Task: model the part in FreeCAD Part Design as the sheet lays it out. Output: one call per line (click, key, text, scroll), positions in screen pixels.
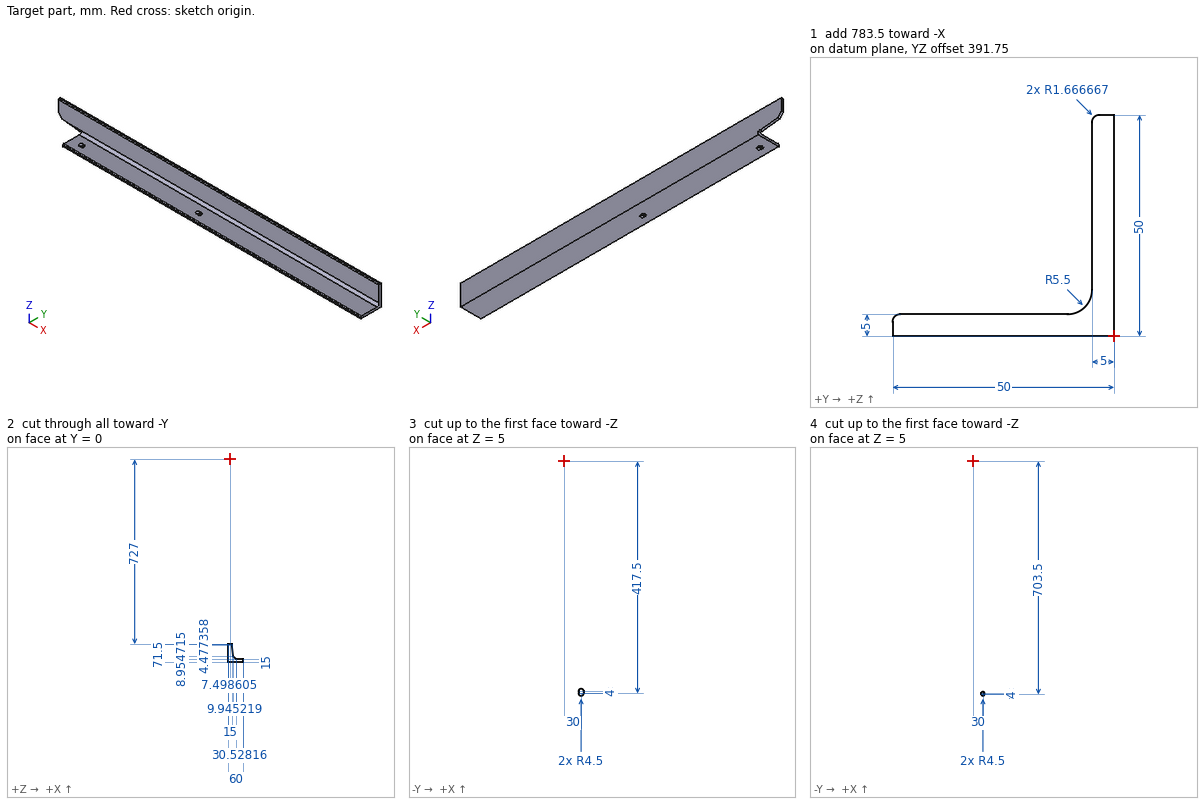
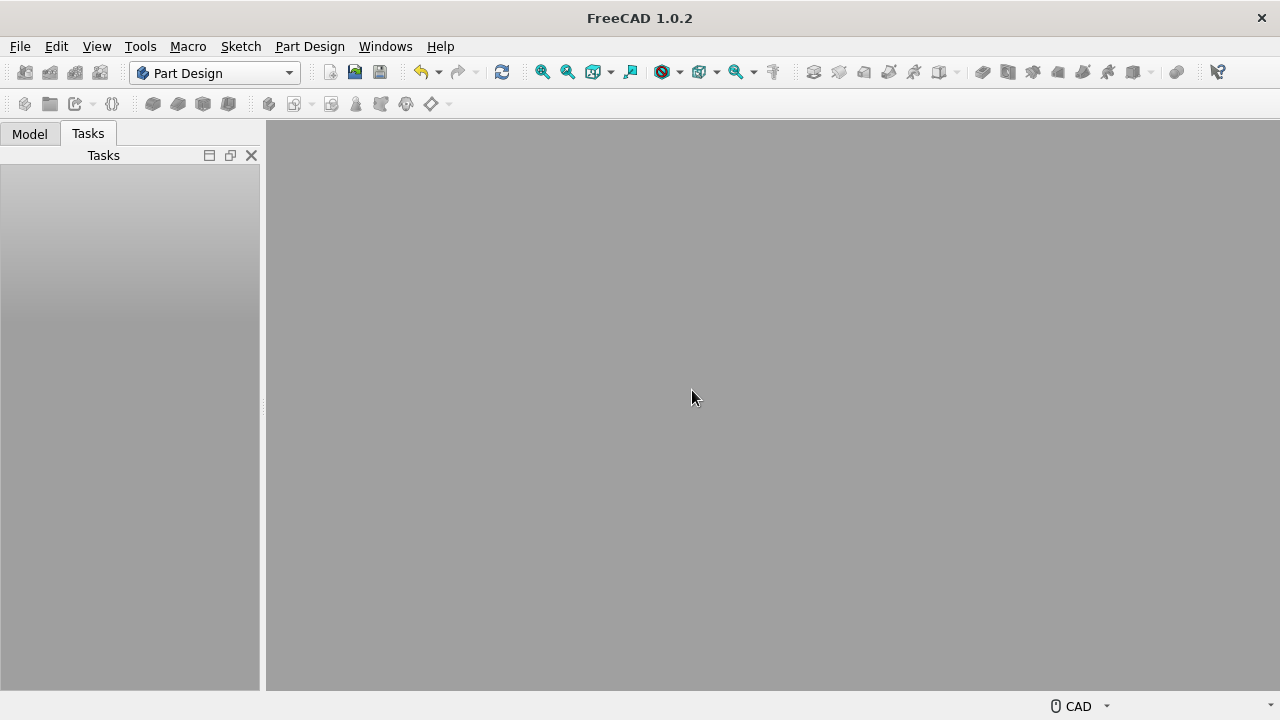
key(ctrl+n)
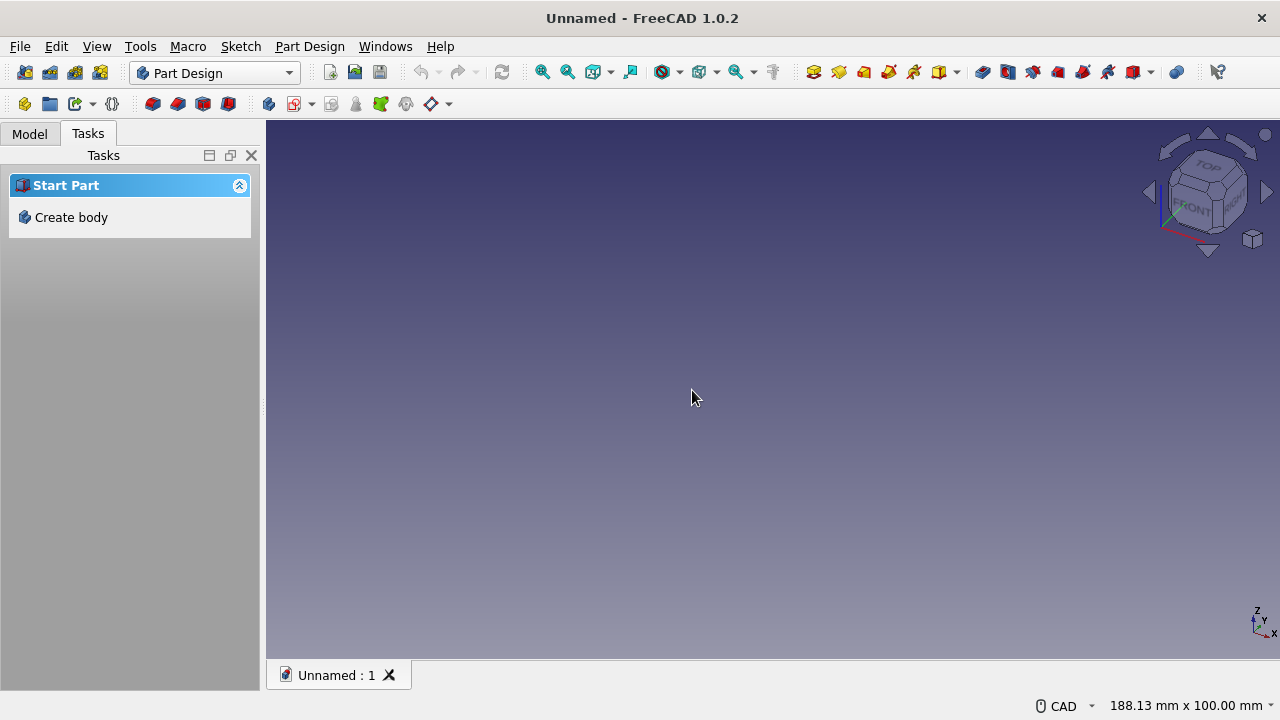
click(269, 104)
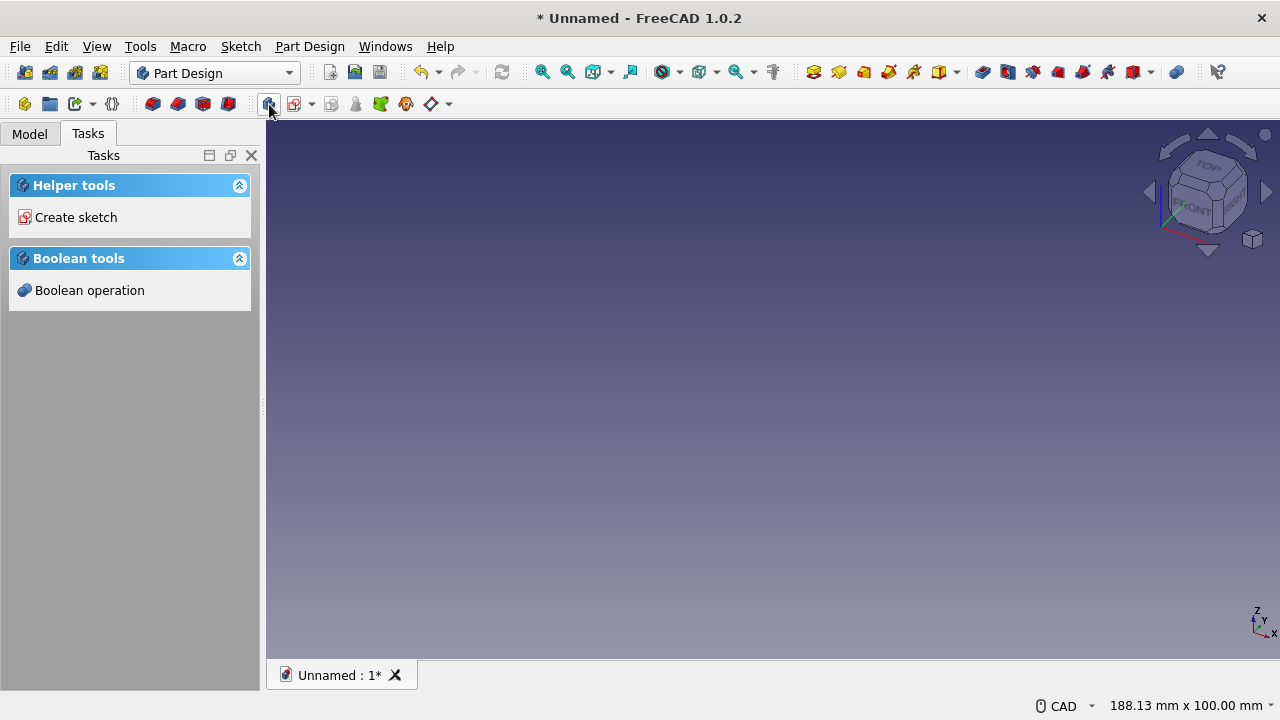
click(30, 134)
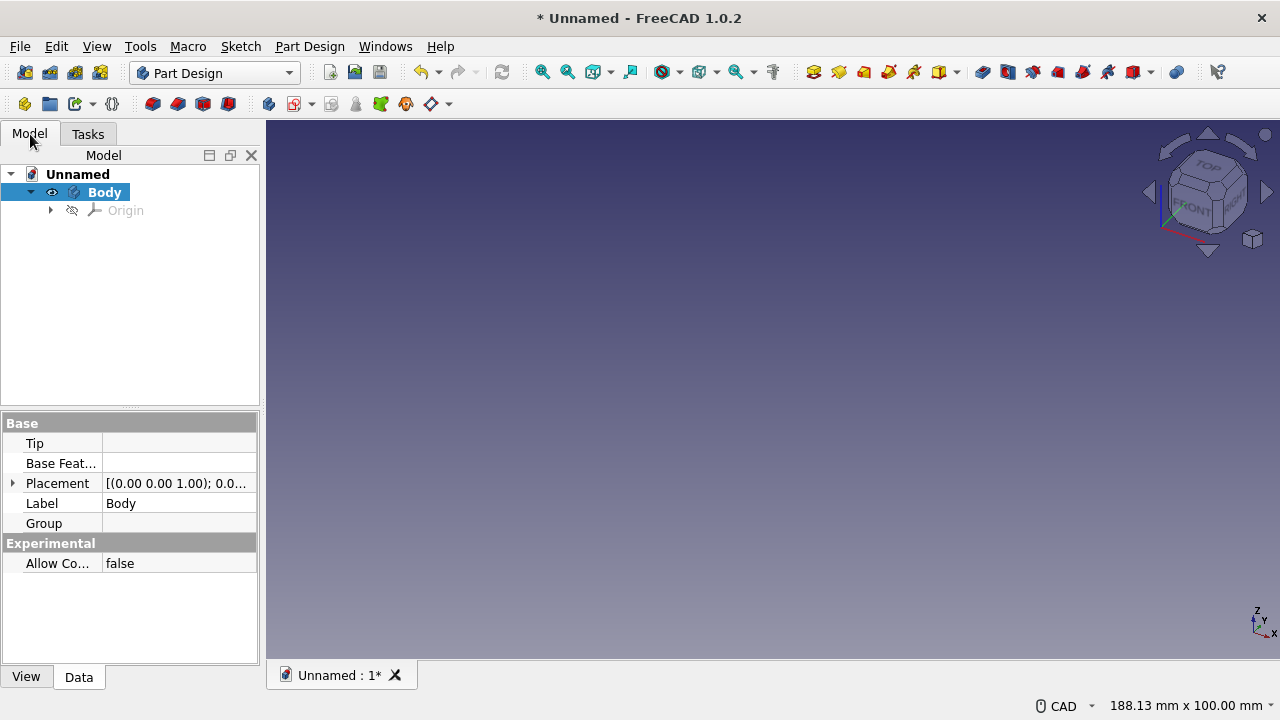
click(51, 210)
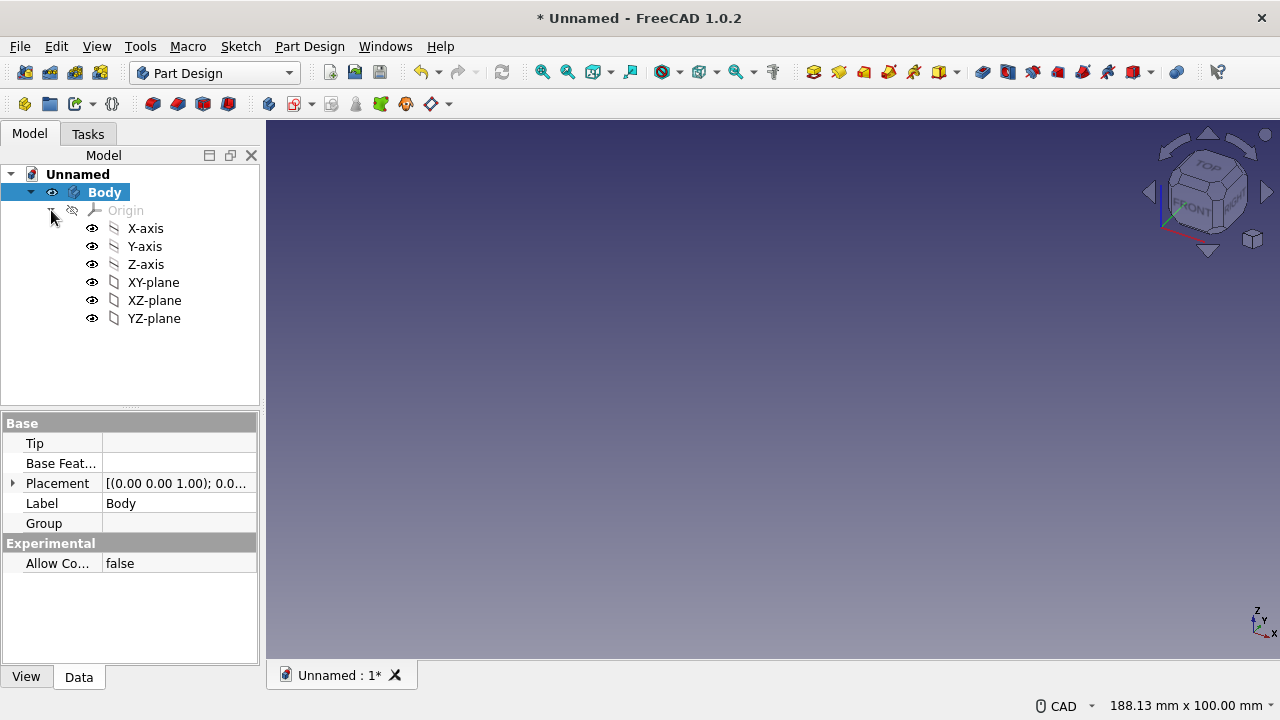
click(137, 318)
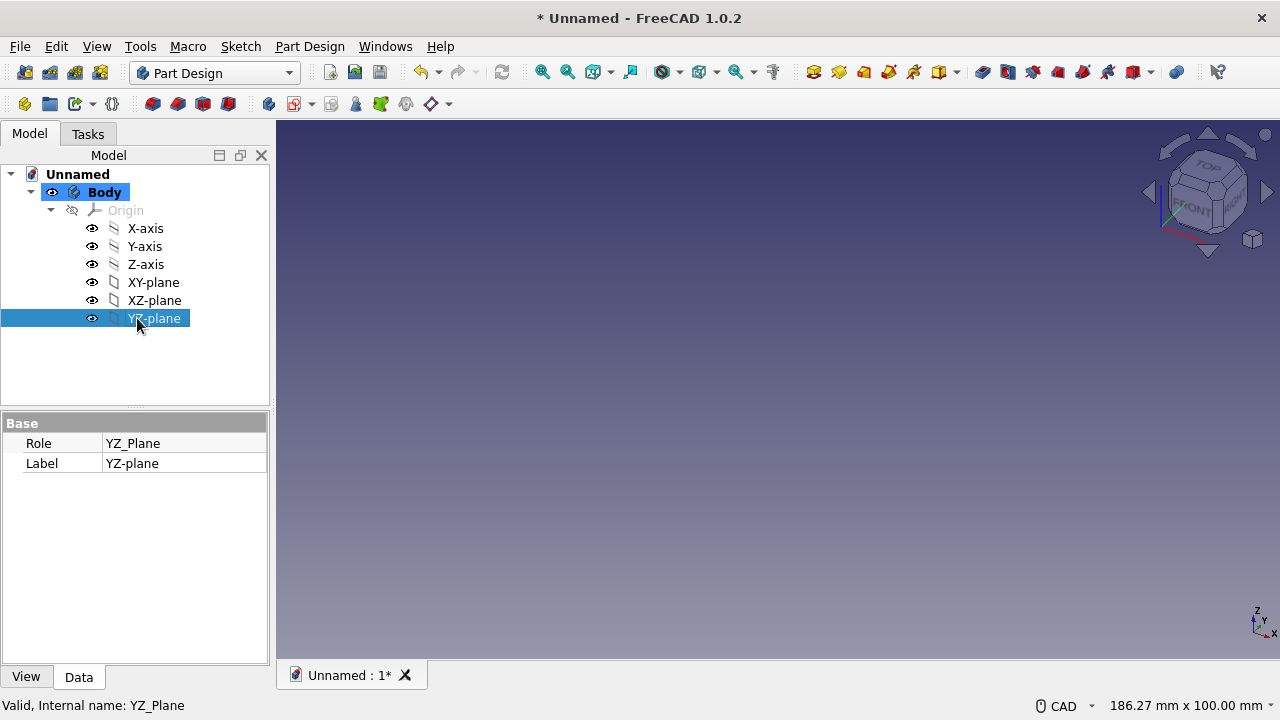
click(430, 104)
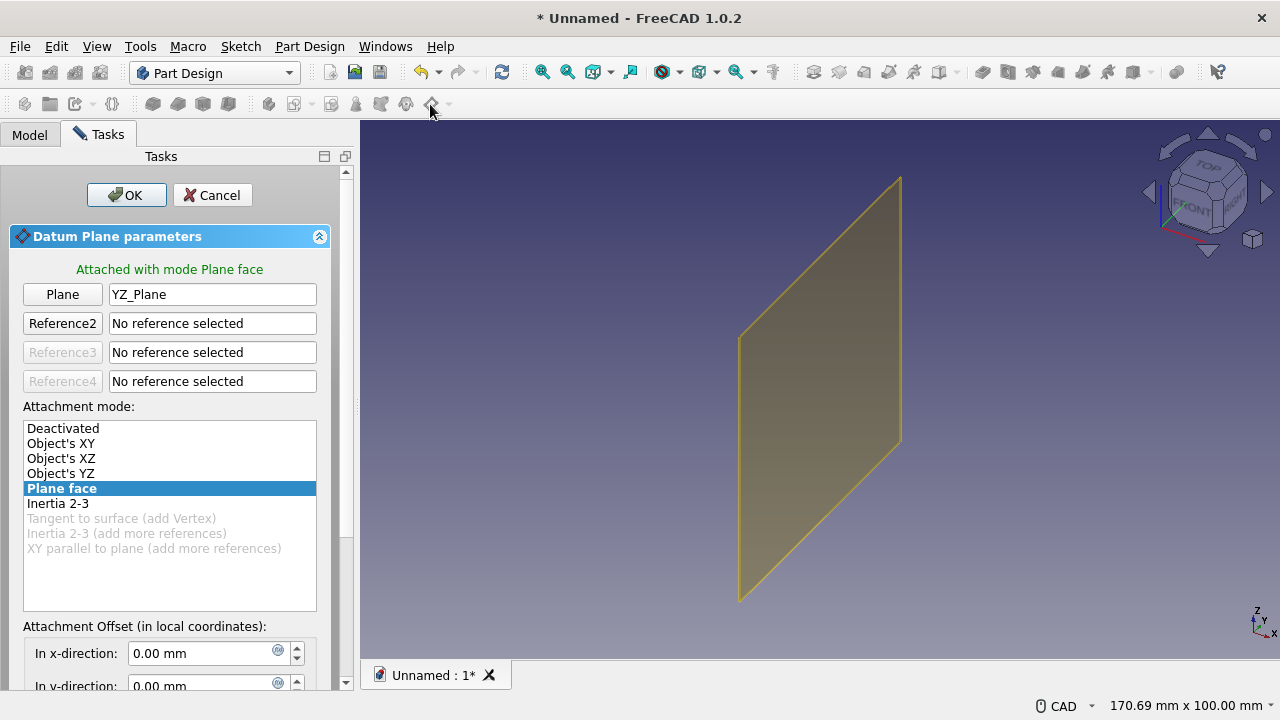
scroll(346, 428, down, 2)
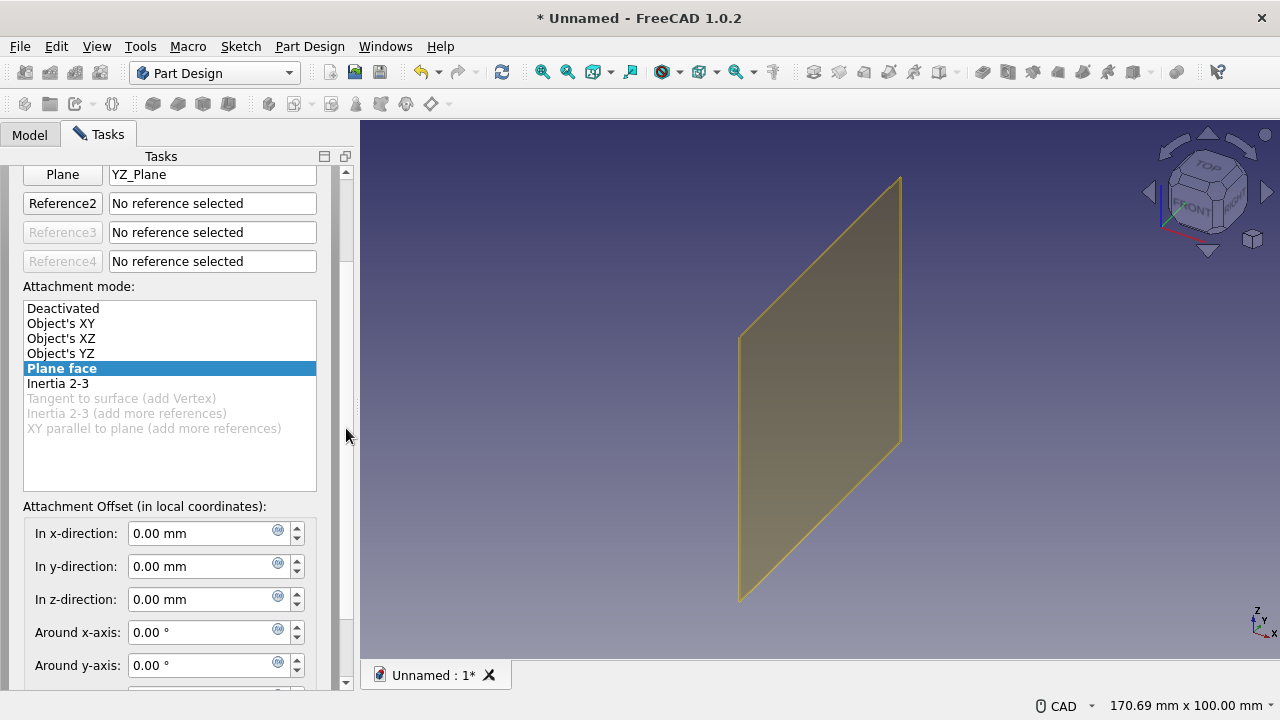
triple_click(210, 600)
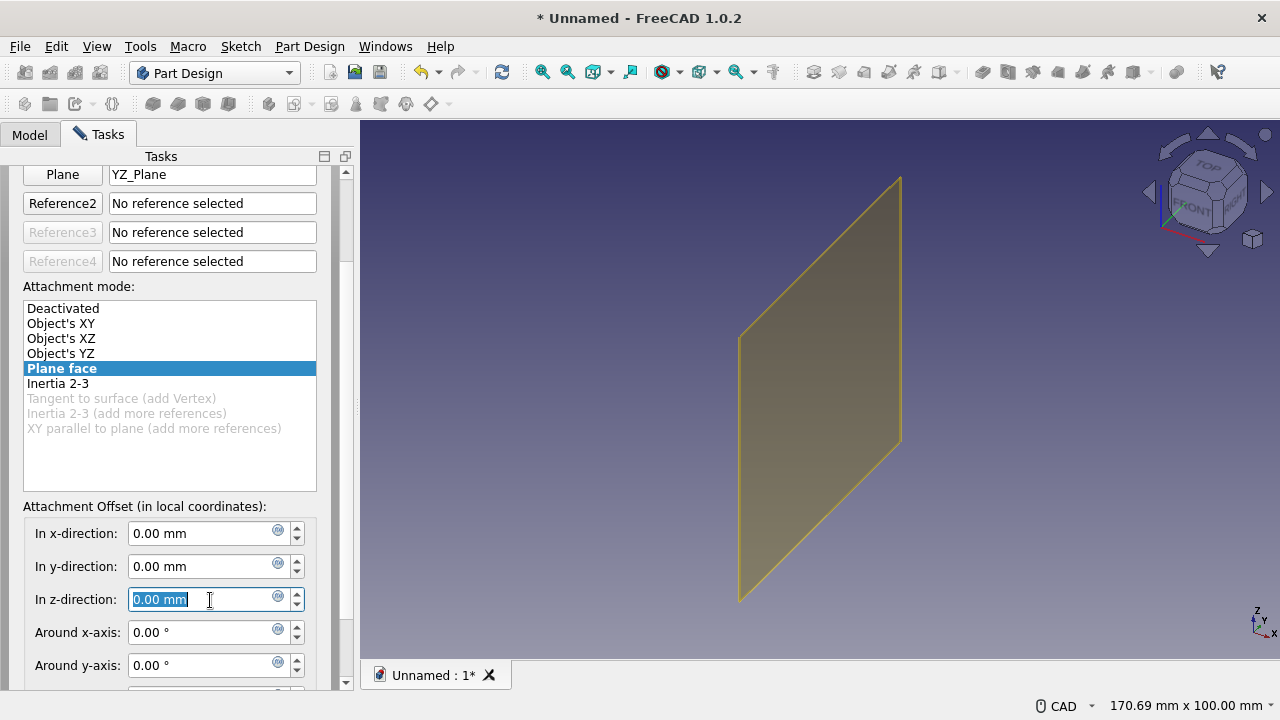
text(391.75)
key(Tab)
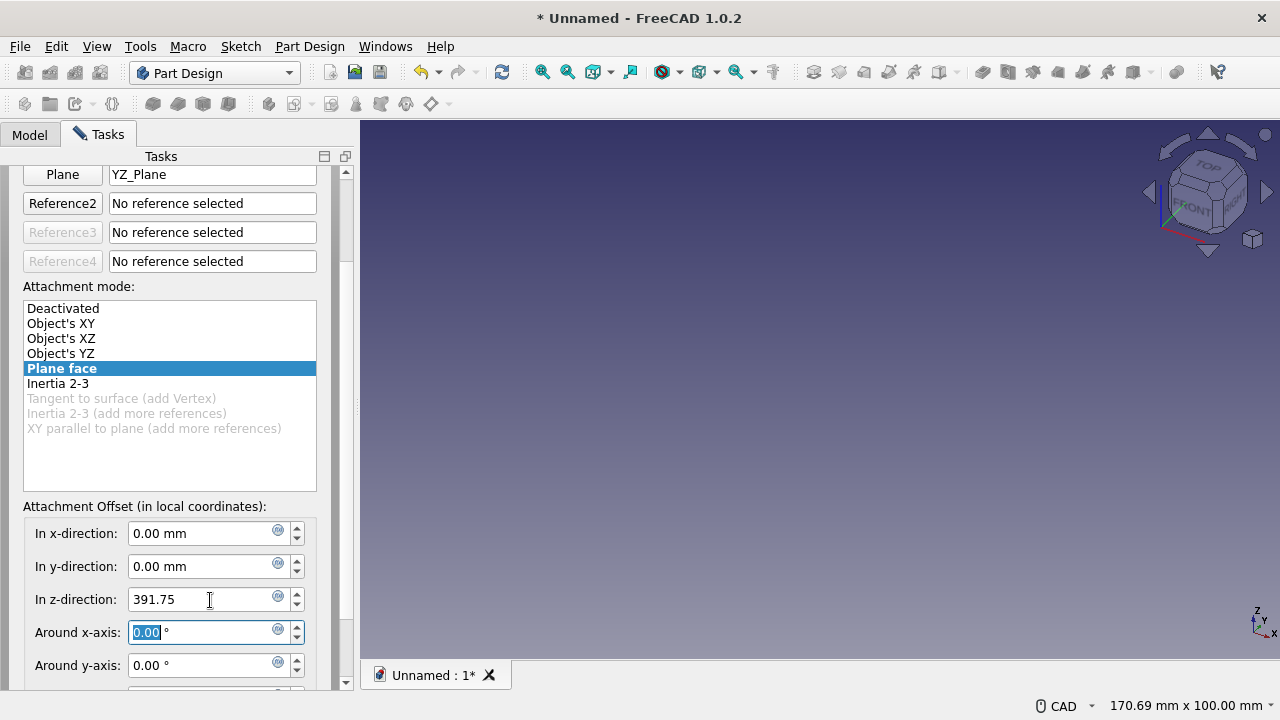
scroll(346, 428, up, 3)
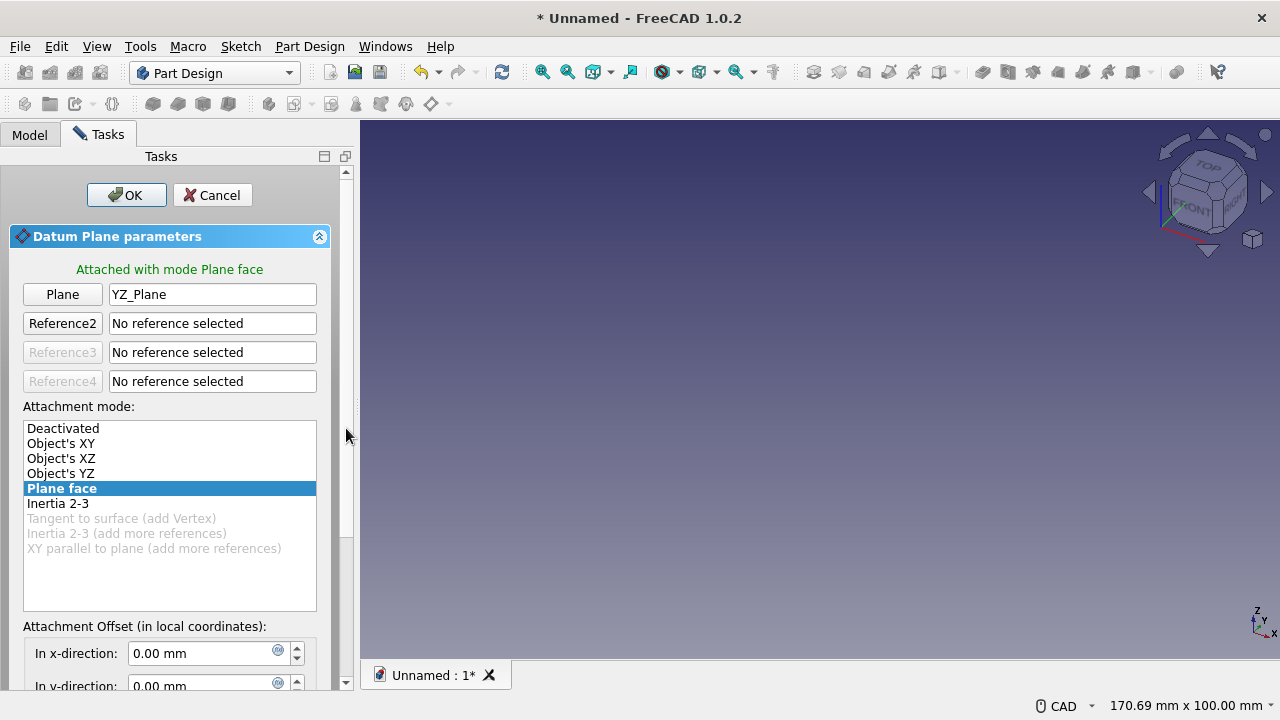
click(127, 195)